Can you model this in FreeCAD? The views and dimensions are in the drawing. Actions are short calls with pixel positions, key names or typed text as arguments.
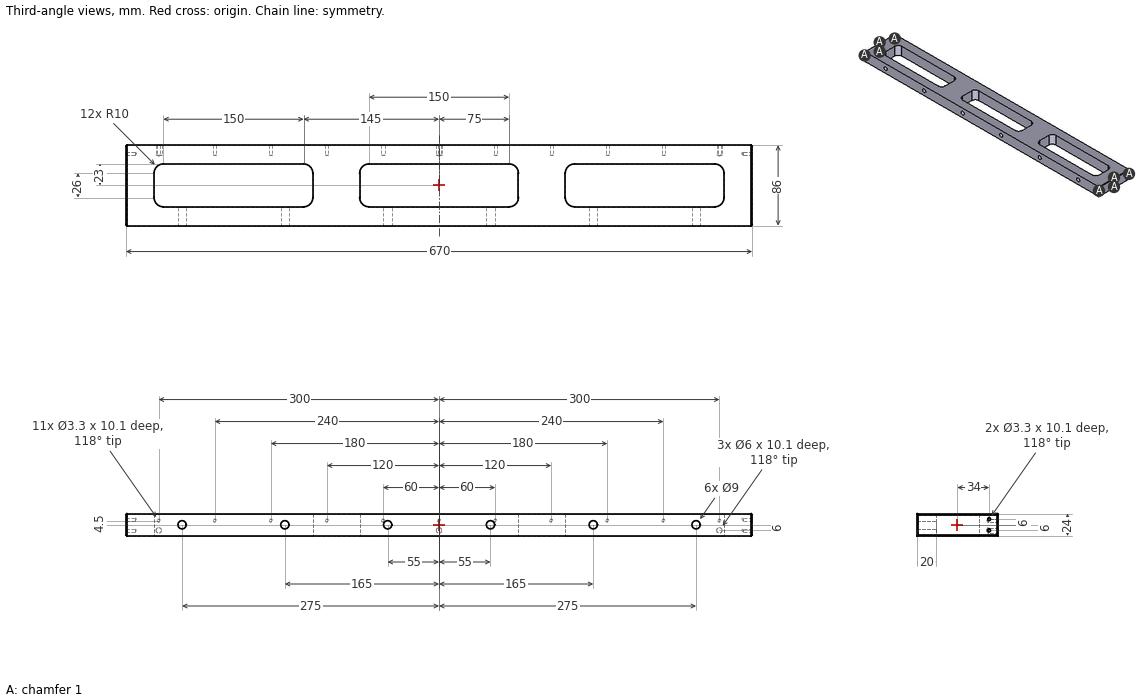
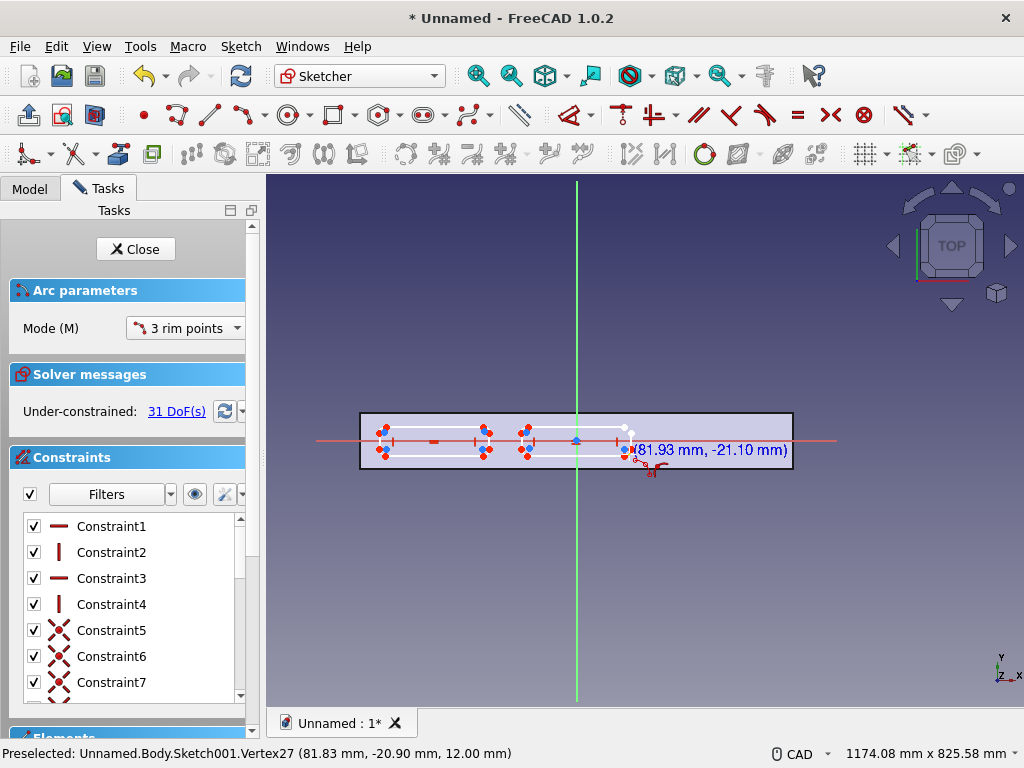
scroll(631, 433, up, 4)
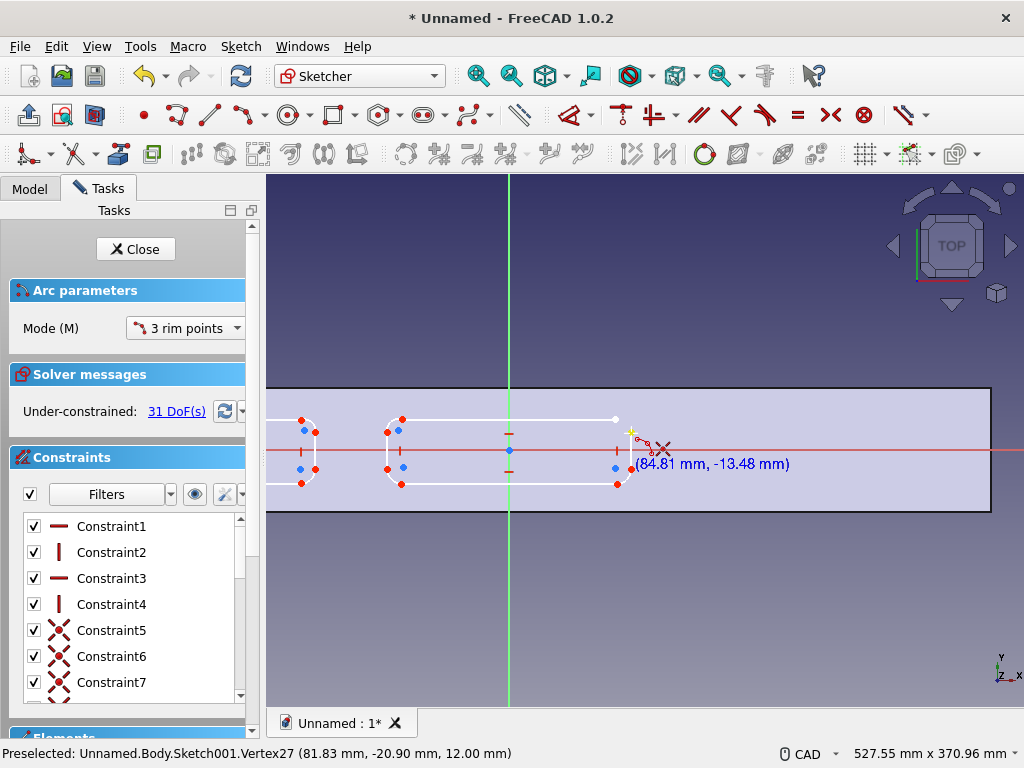
click(631, 432)
click(616, 420)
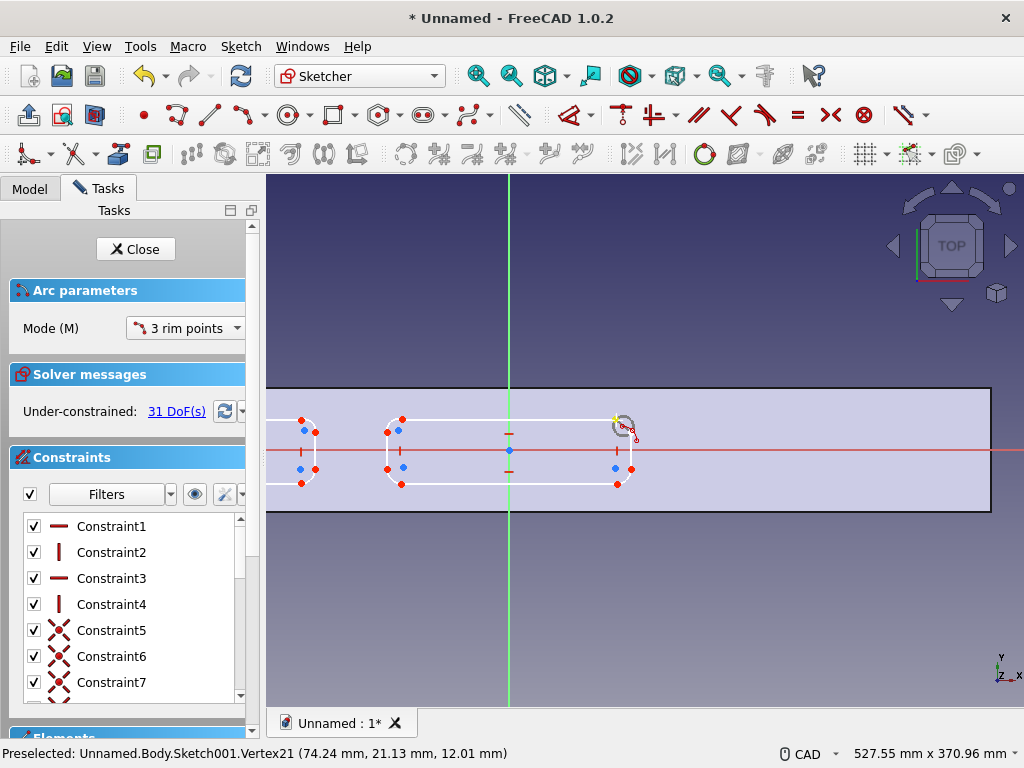
scroll(627, 421, up, 7)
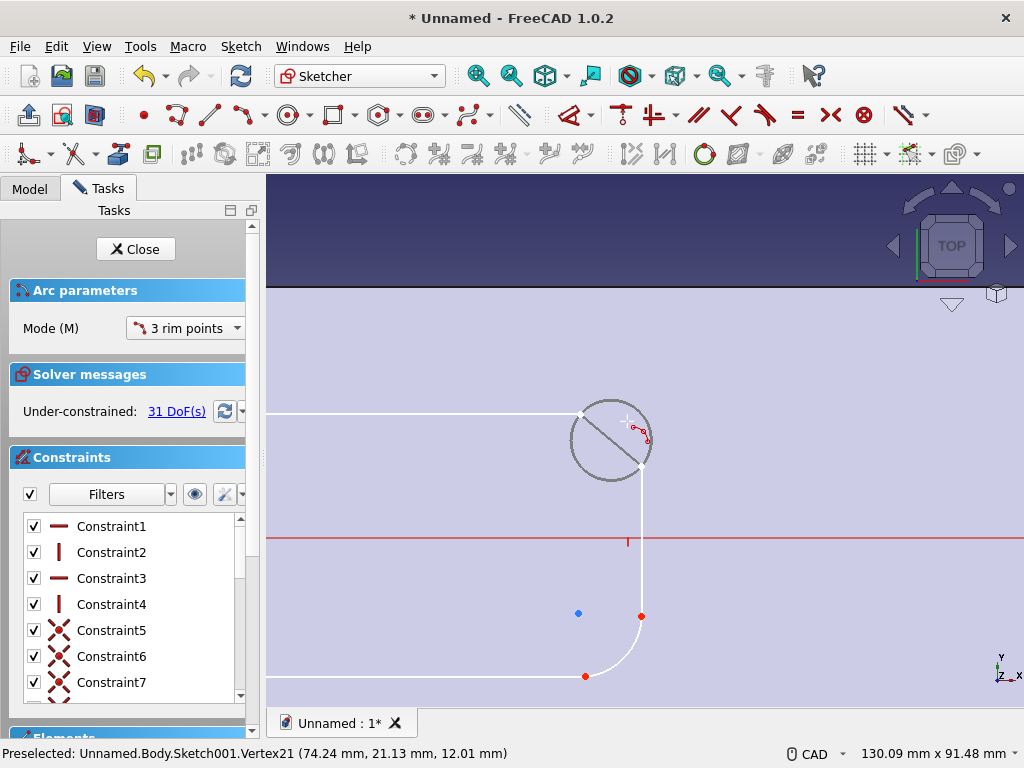
click(626, 421)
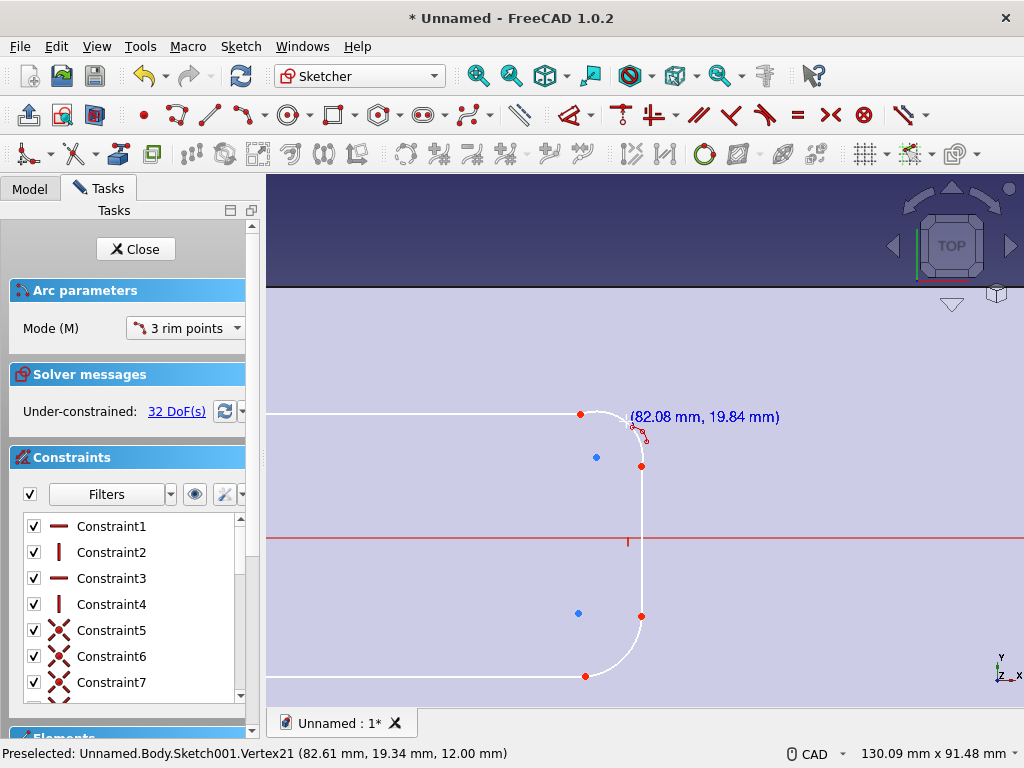
click(210, 116)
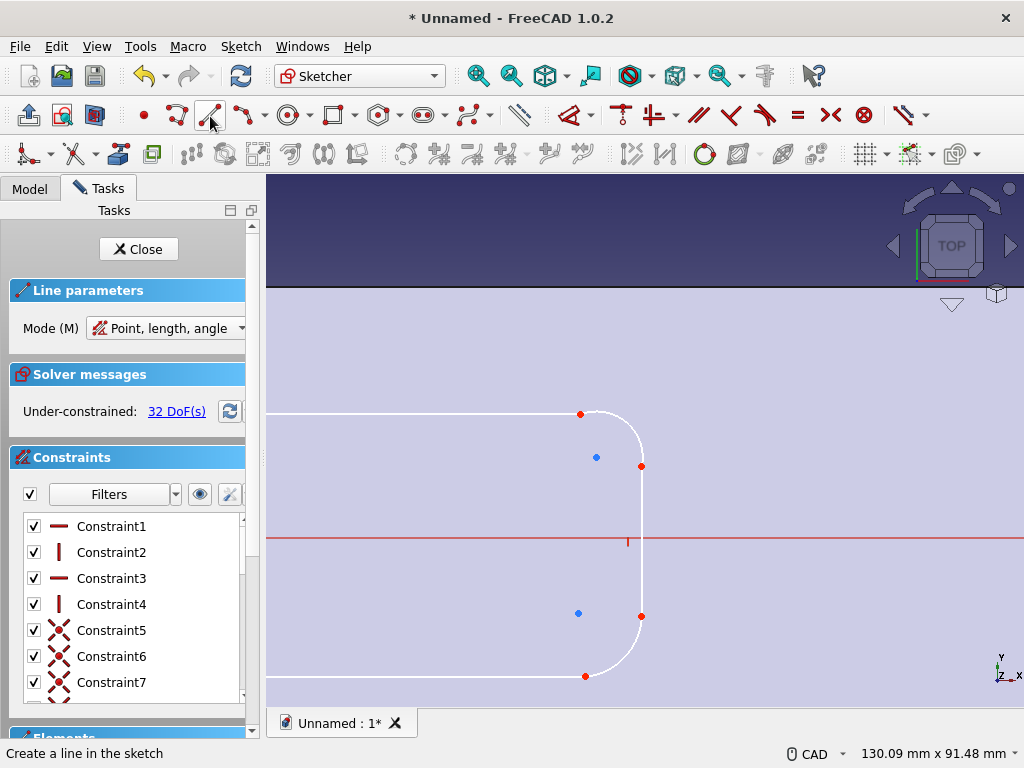
scroll(630, 428, down, 11)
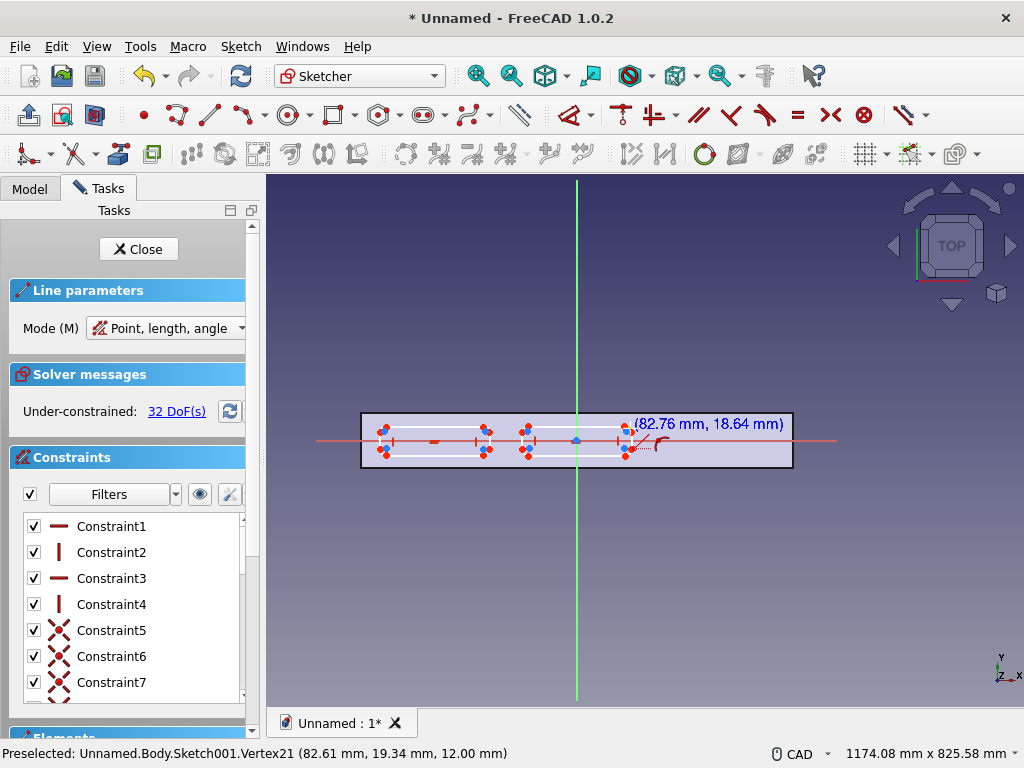
click(767, 426)
click(671, 426)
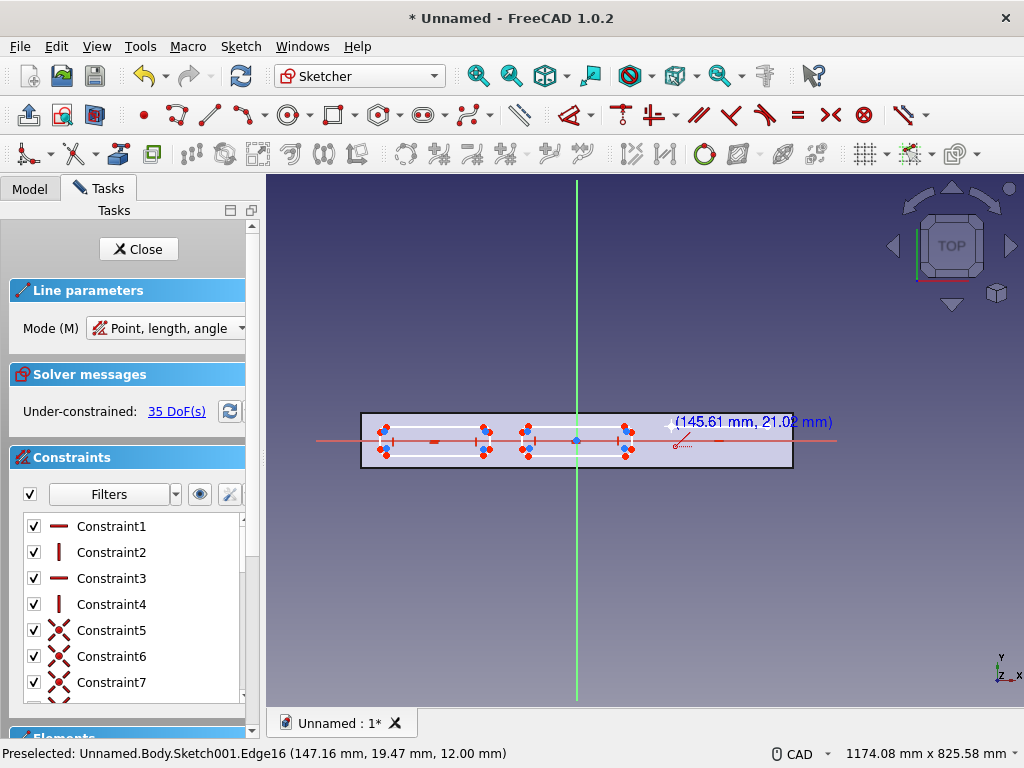
scroll(664, 432, up, 4)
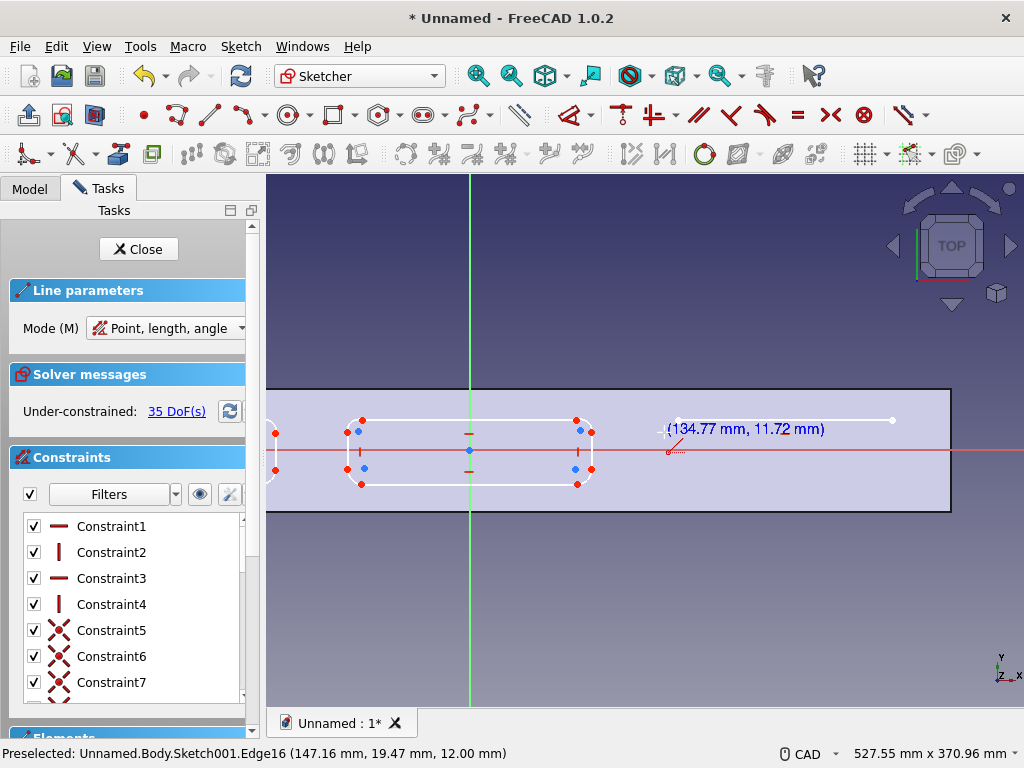
click(664, 432)
click(664, 469)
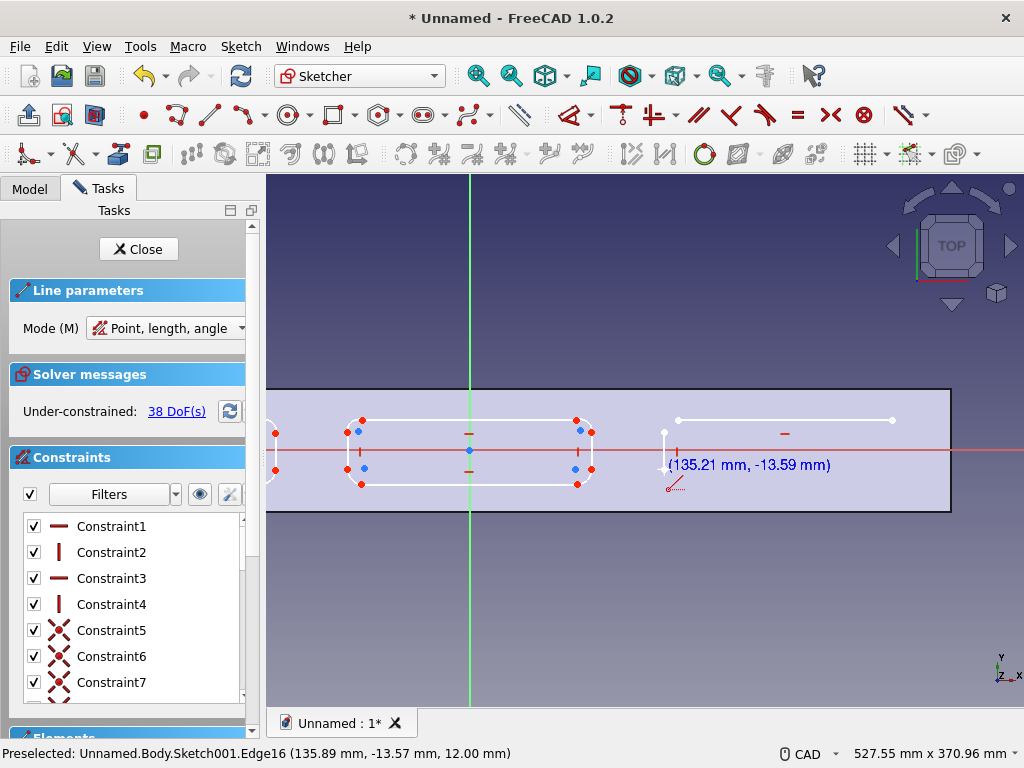
click(678, 484)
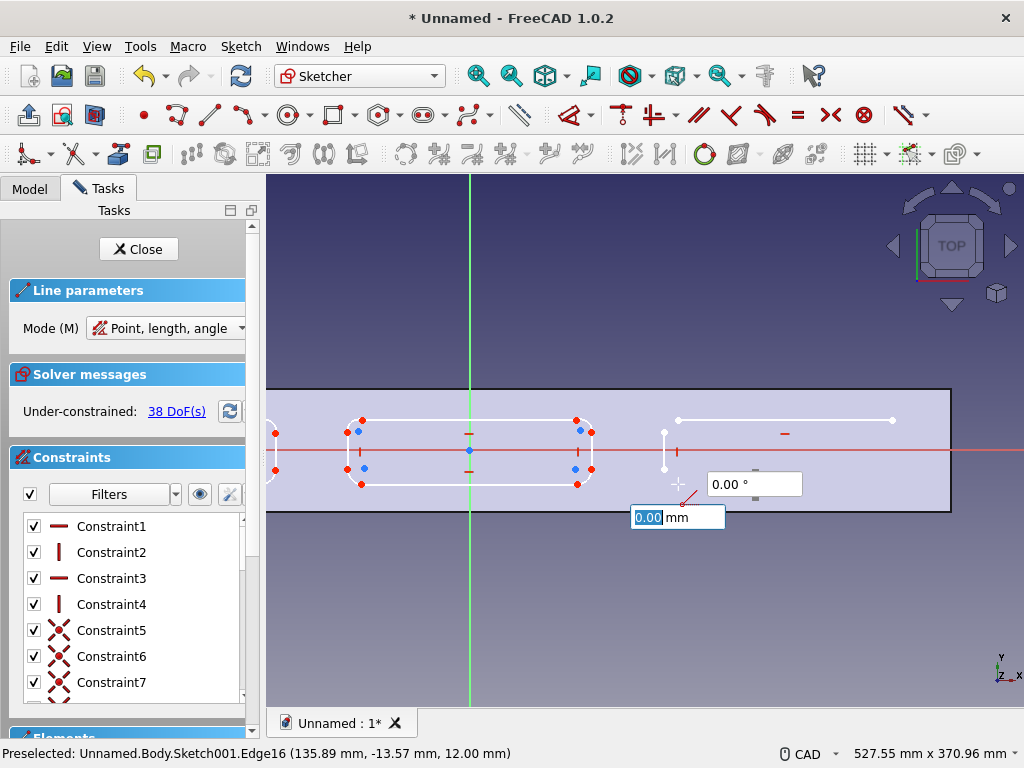
scroll(664, 432, down, 4)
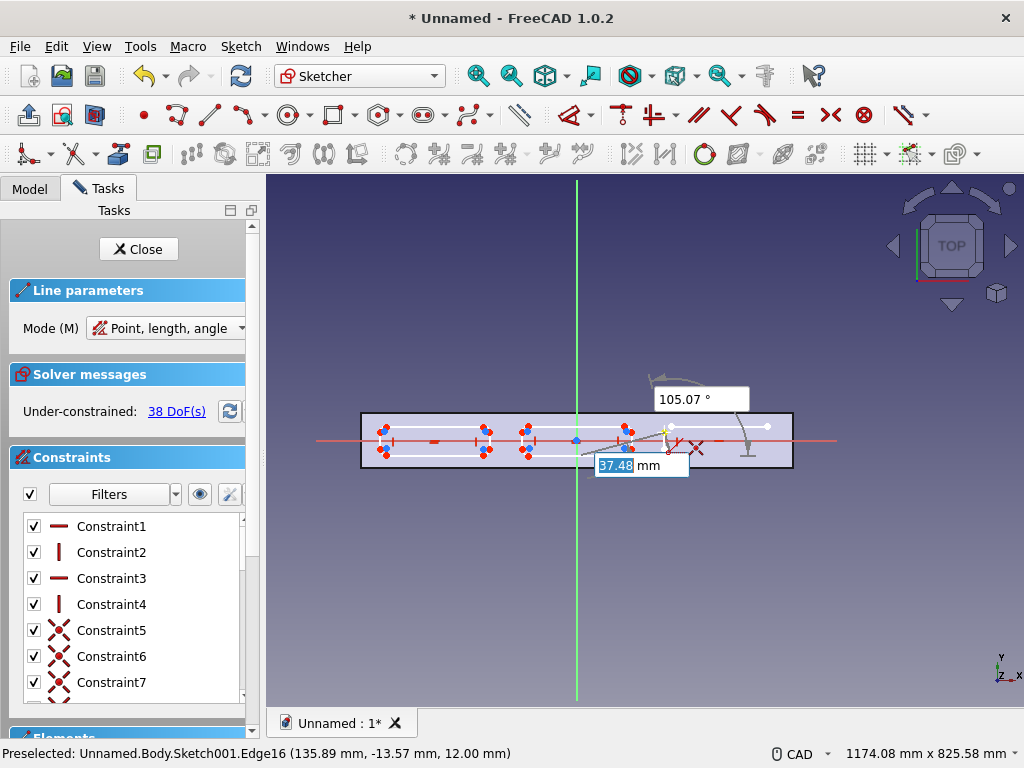
click(767, 456)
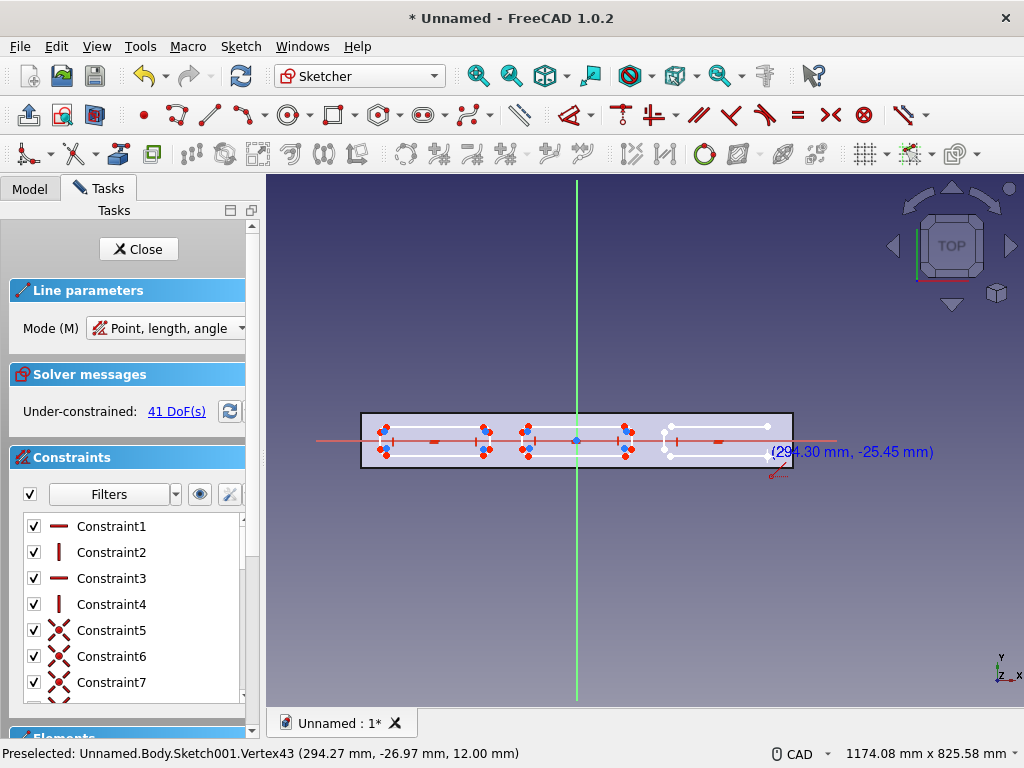
scroll(774, 449, up, 4)